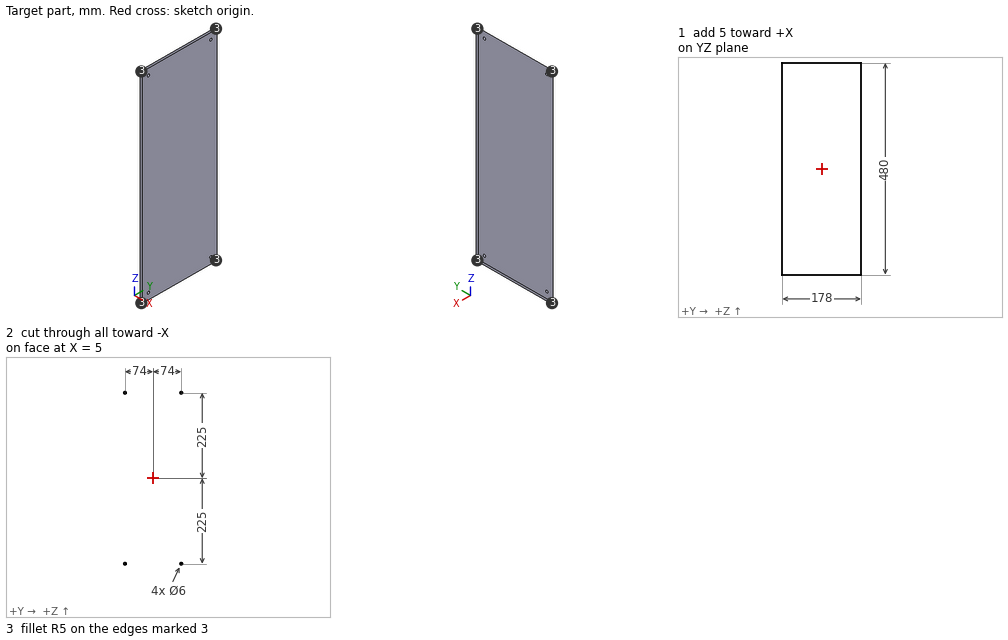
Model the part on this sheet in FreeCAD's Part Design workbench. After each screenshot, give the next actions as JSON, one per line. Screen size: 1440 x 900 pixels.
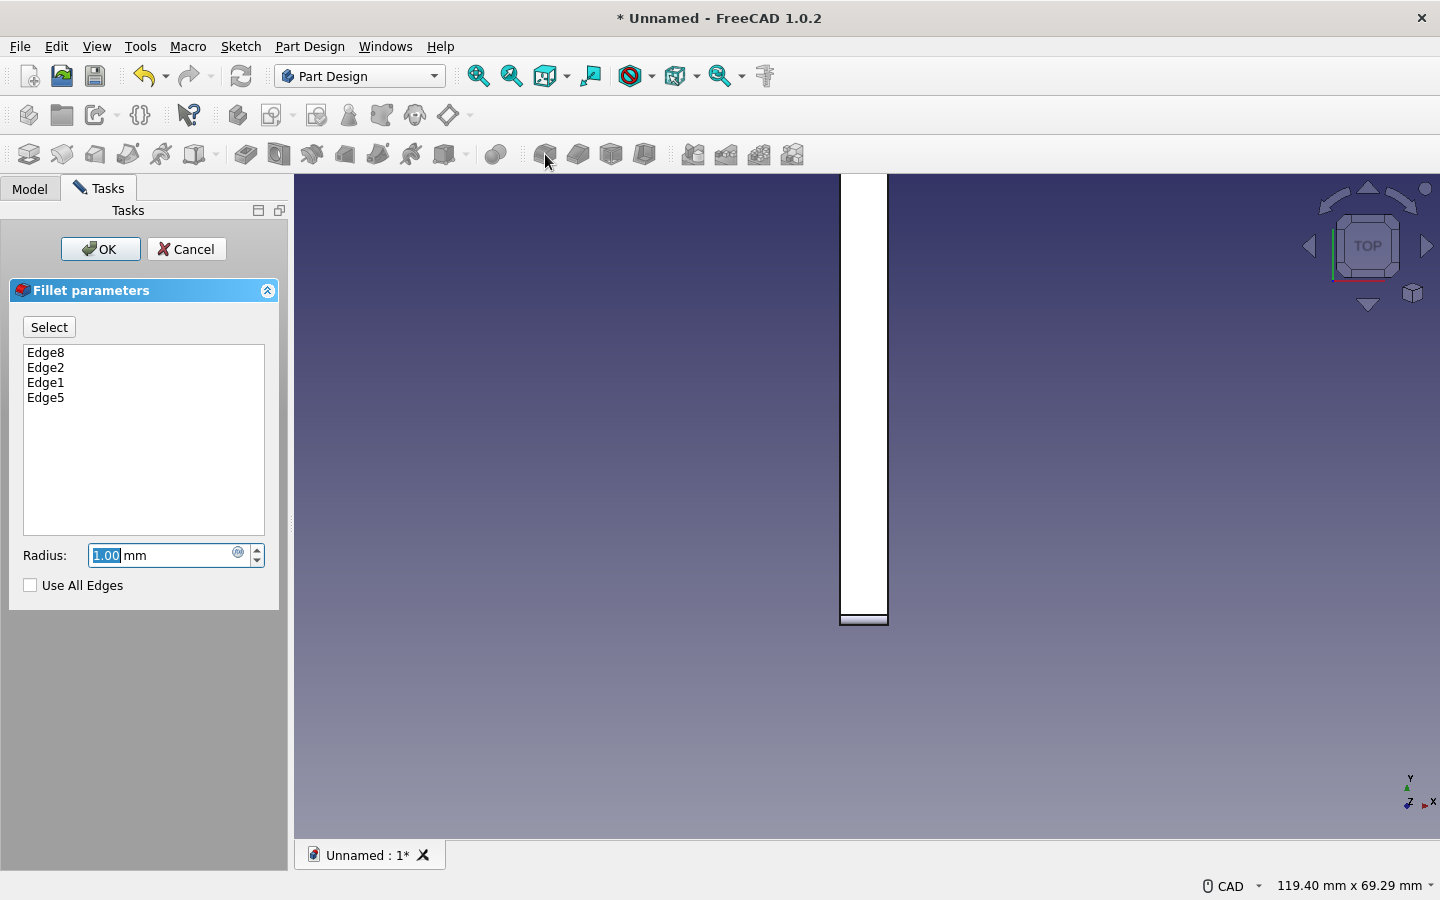
{"action": "type", "text": "5"}
{"action": "key", "text": "Tab"}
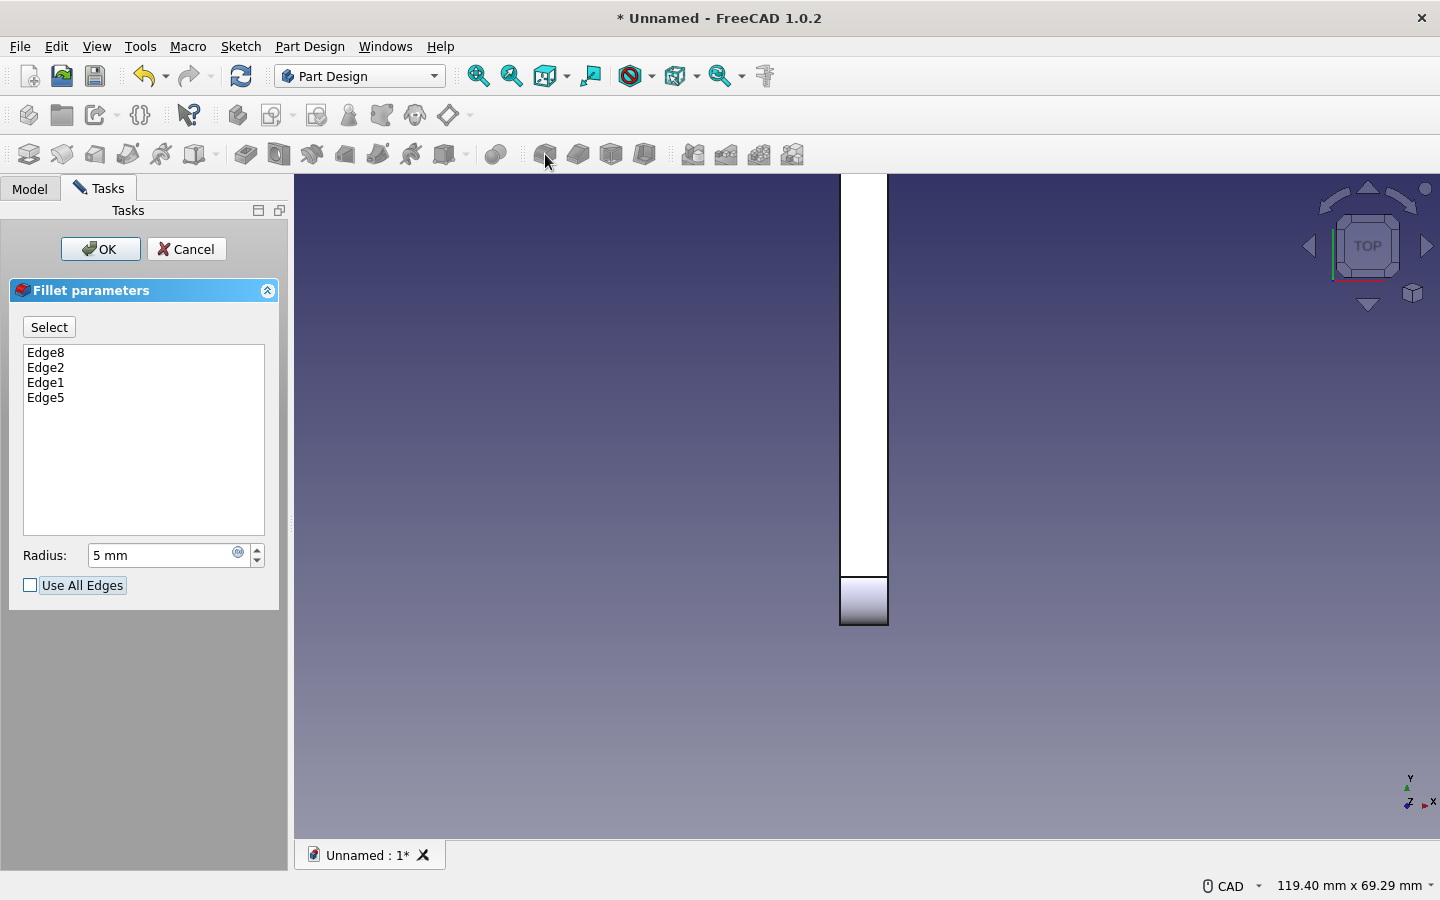
{"action": "left_click", "coordinate": [101, 249]}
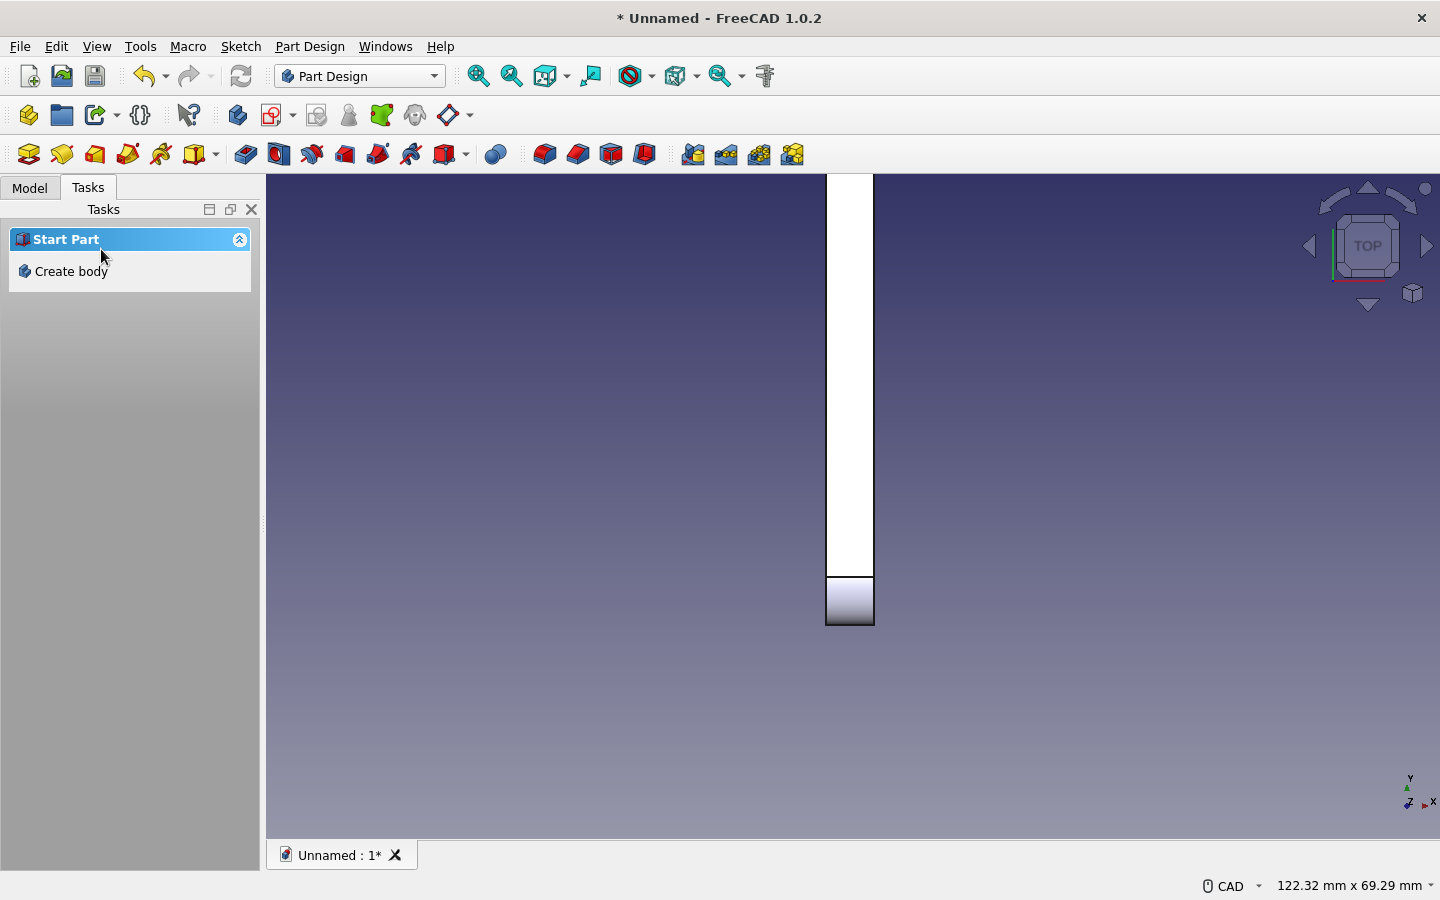
{"action": "key", "text": "0"}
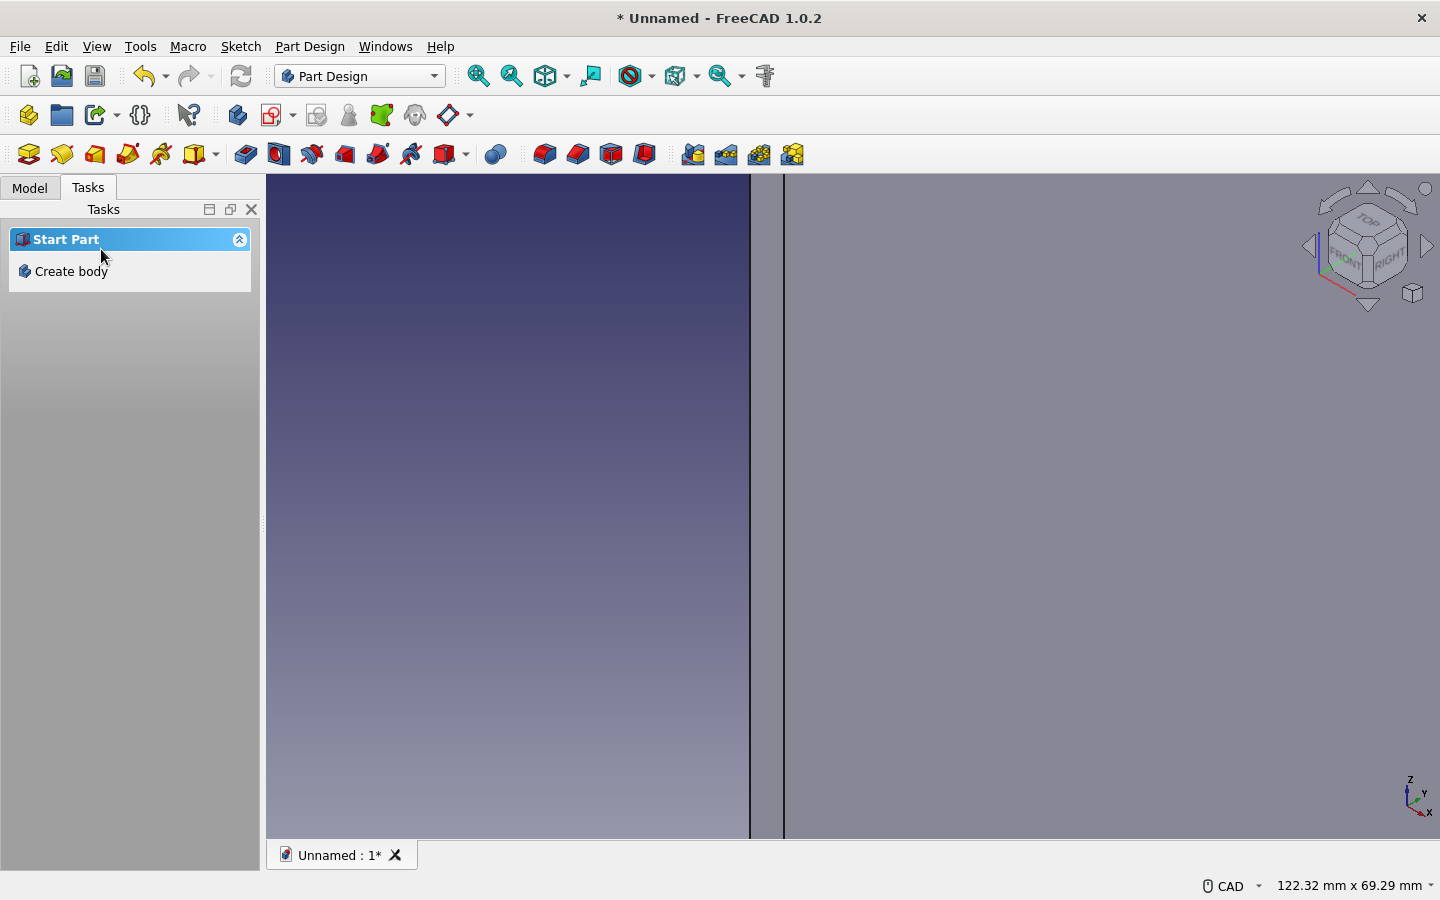
{"action": "left_click", "coordinate": [479, 76]}